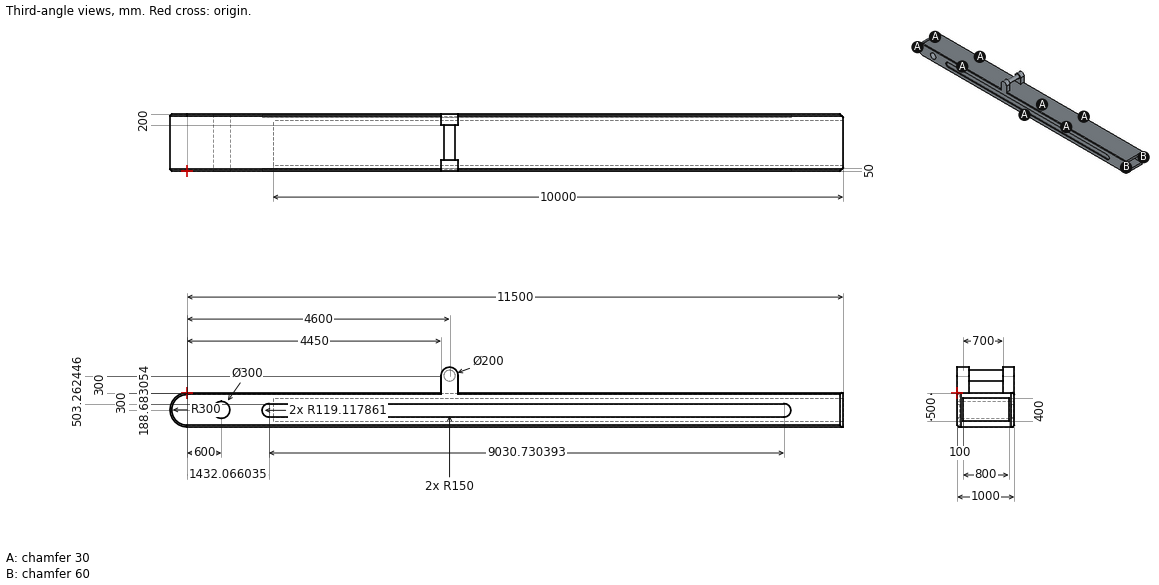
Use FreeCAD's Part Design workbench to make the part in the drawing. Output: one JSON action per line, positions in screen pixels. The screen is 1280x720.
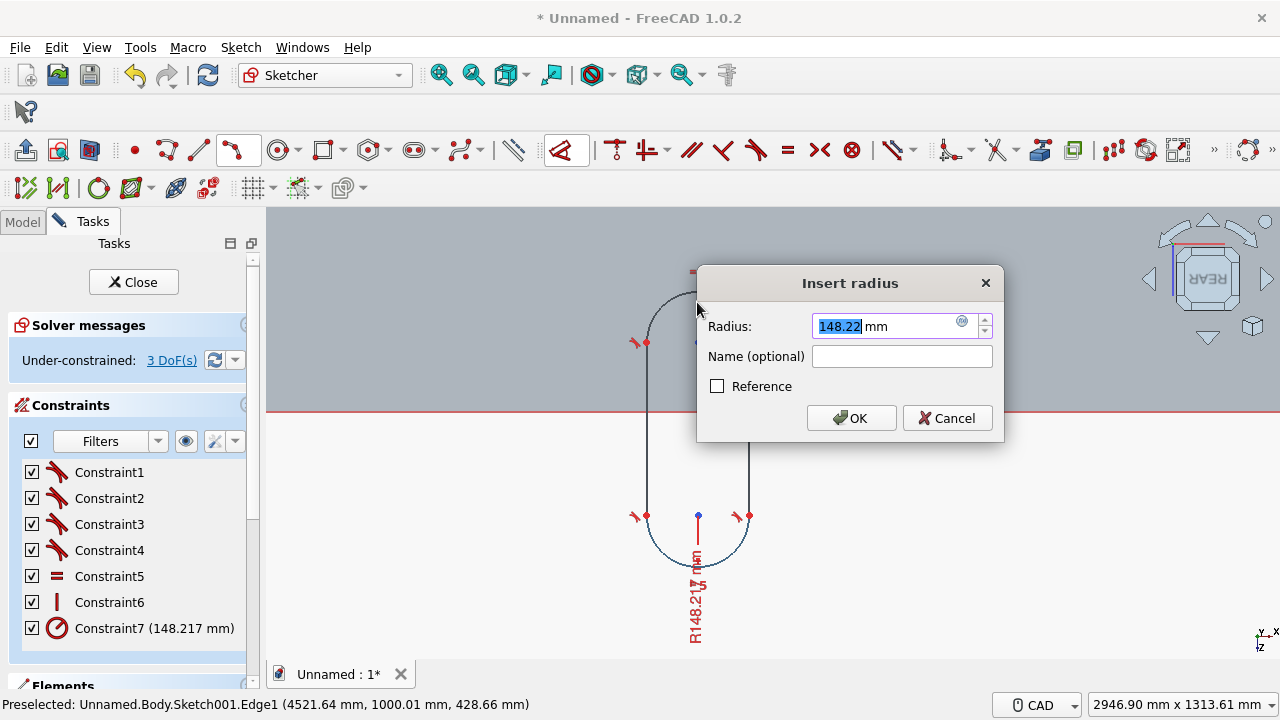
{"action": "type", "text": "150"}
{"action": "key", "text": "Return"}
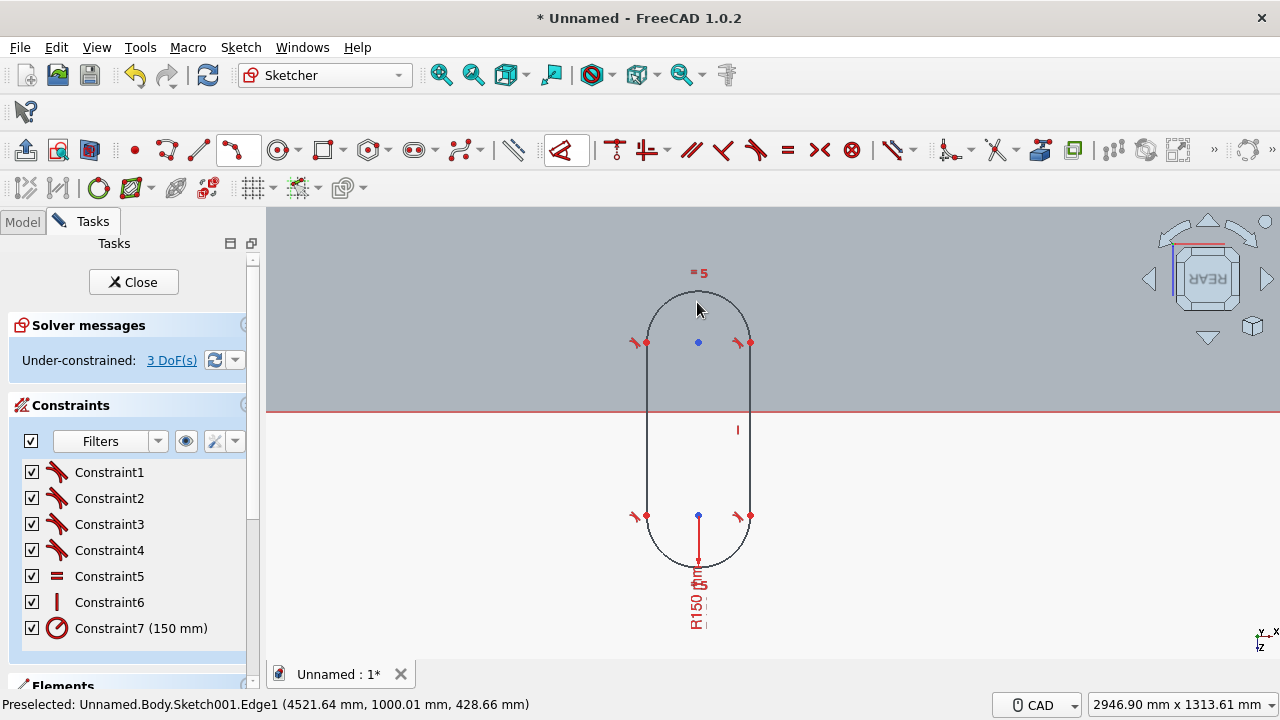
{"action": "left_click", "coordinate": [647, 516]}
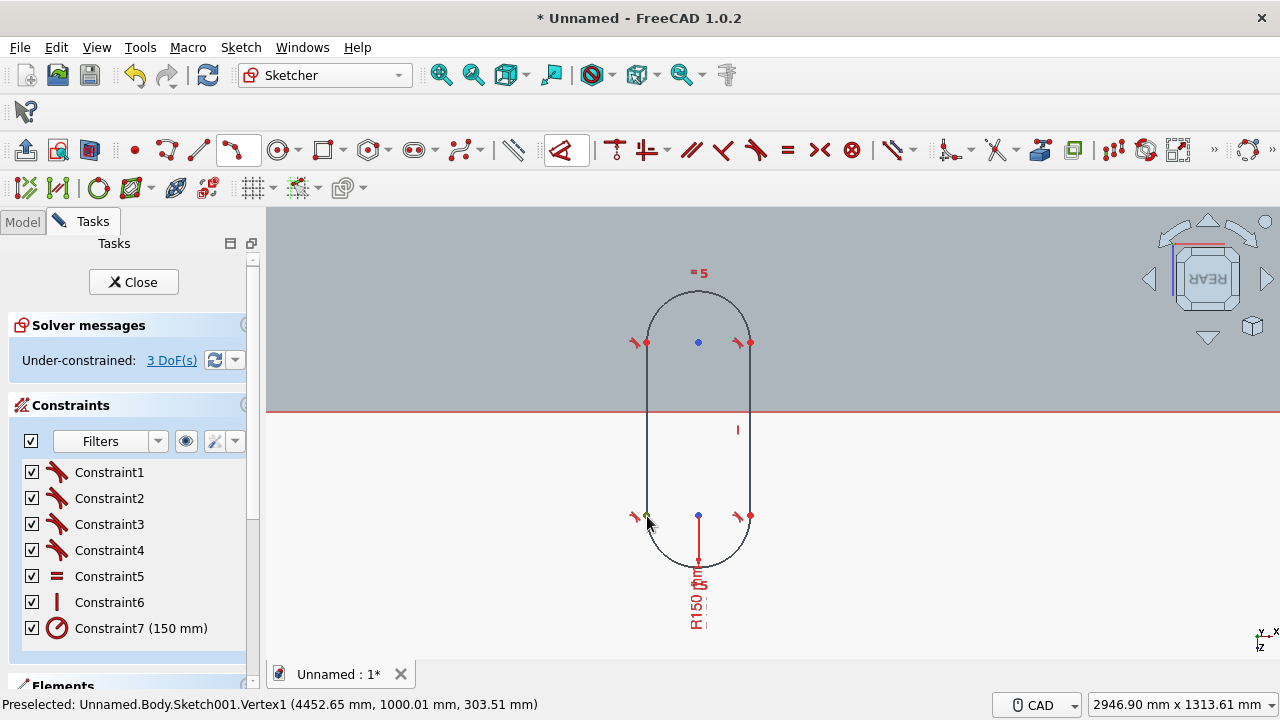
{"action": "left_click", "coordinate": [584, 150]}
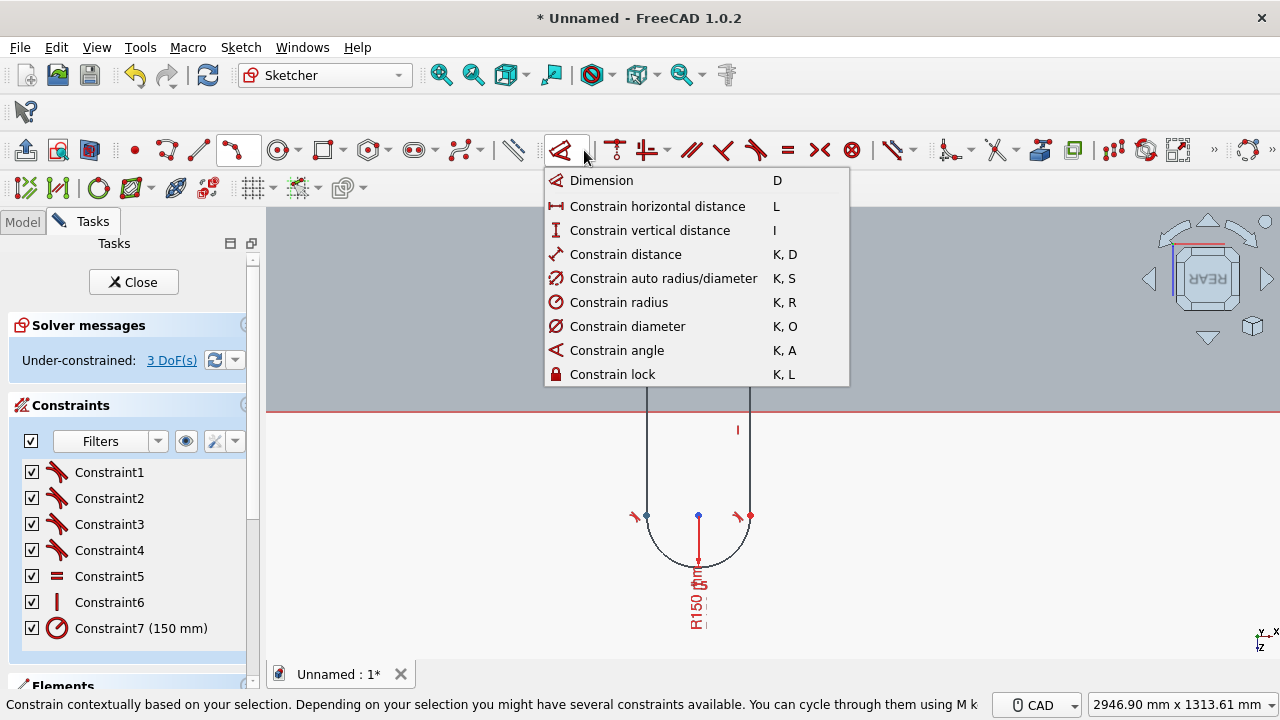
{"action": "left_click", "coordinate": [697, 230]}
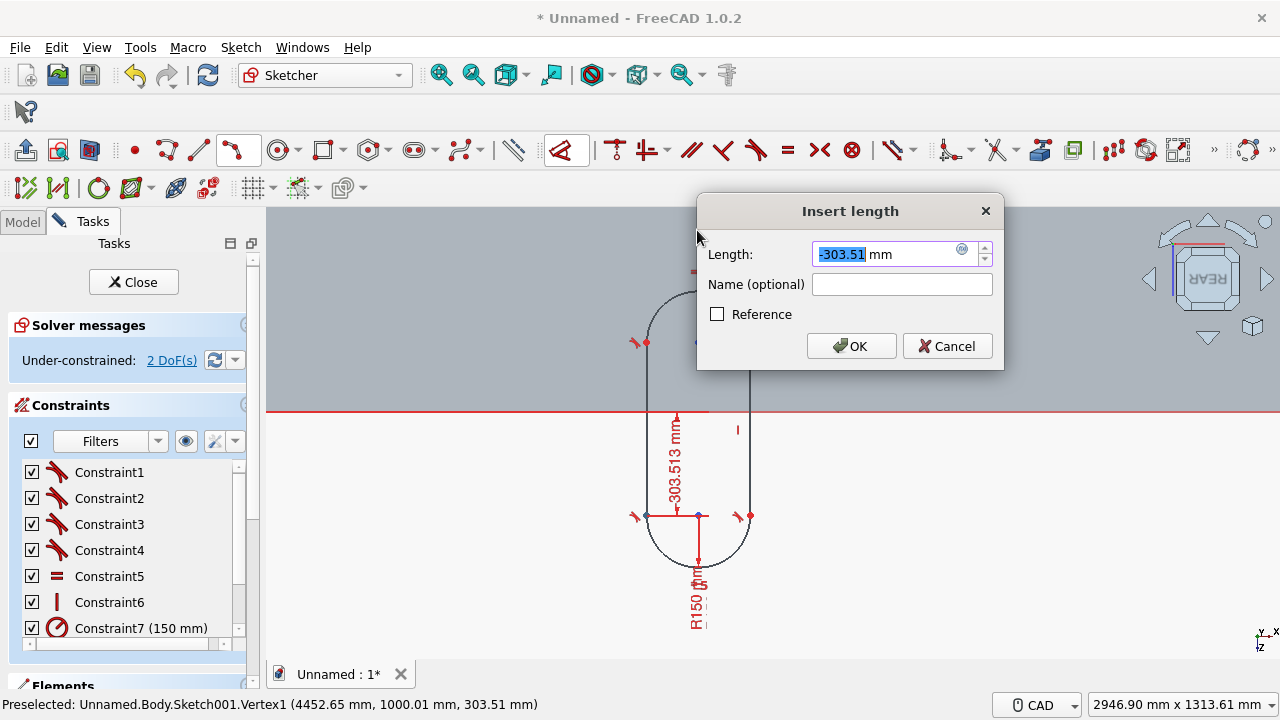
{"action": "type", "text": "-300"}
{"action": "key", "text": "Return"}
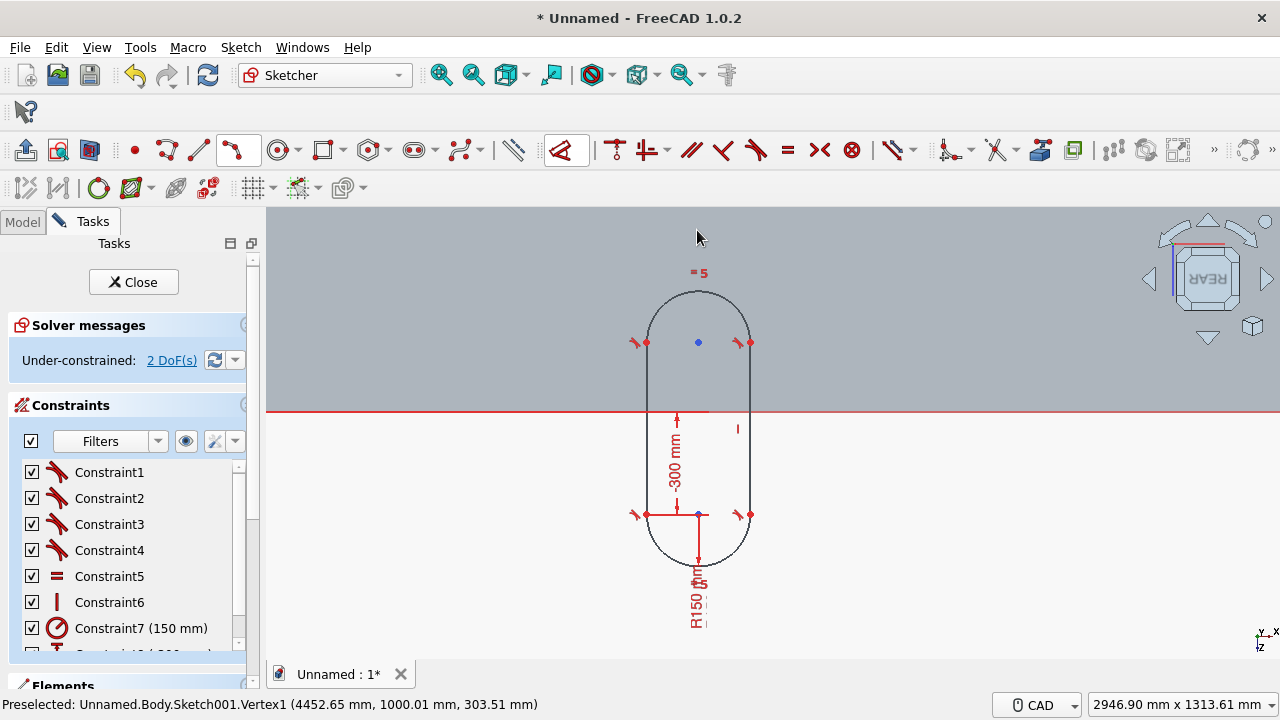
{"action": "left_click", "coordinate": [647, 515]}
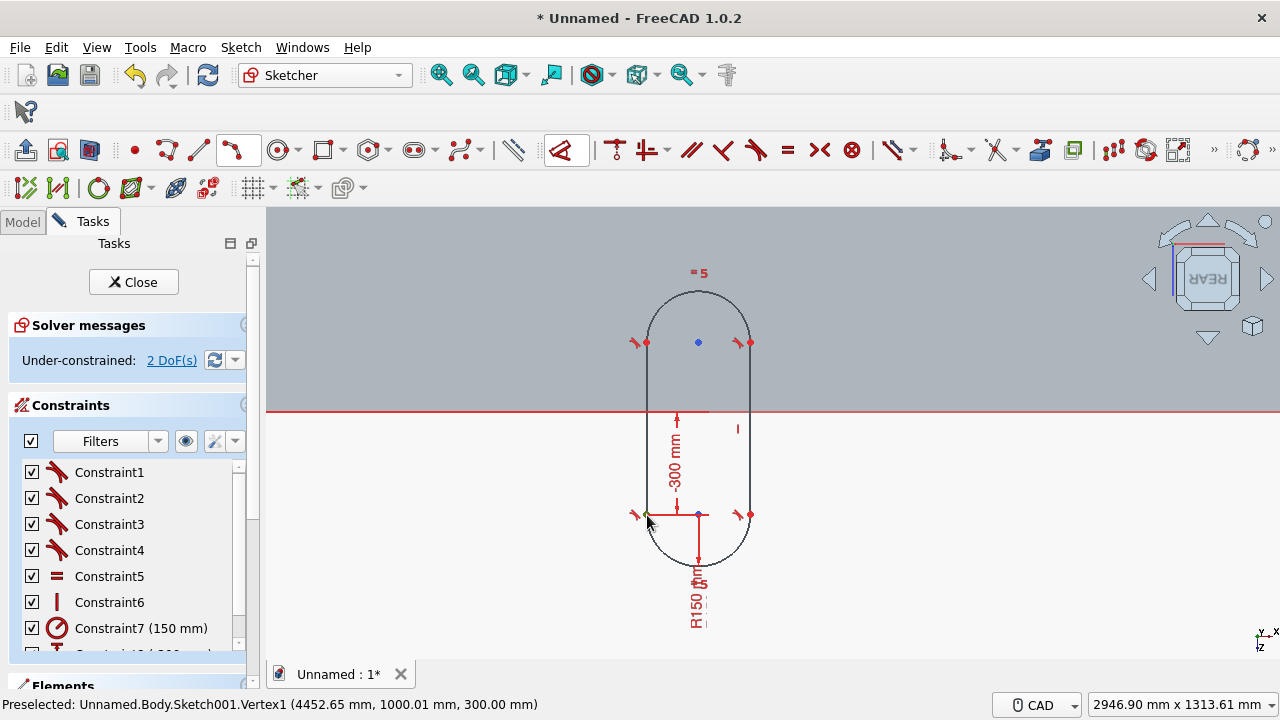
{"action": "key", "text": "l"}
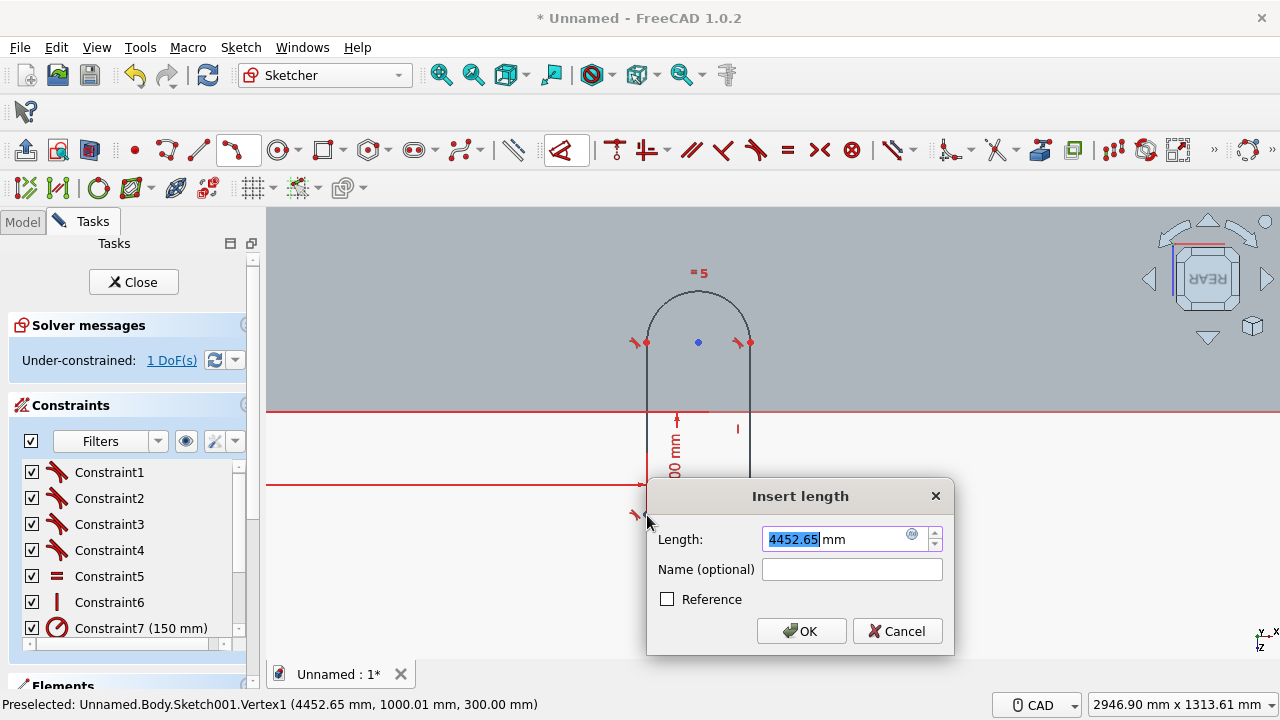
{"action": "type", "text": "4450"}
{"action": "key", "text": "Return"}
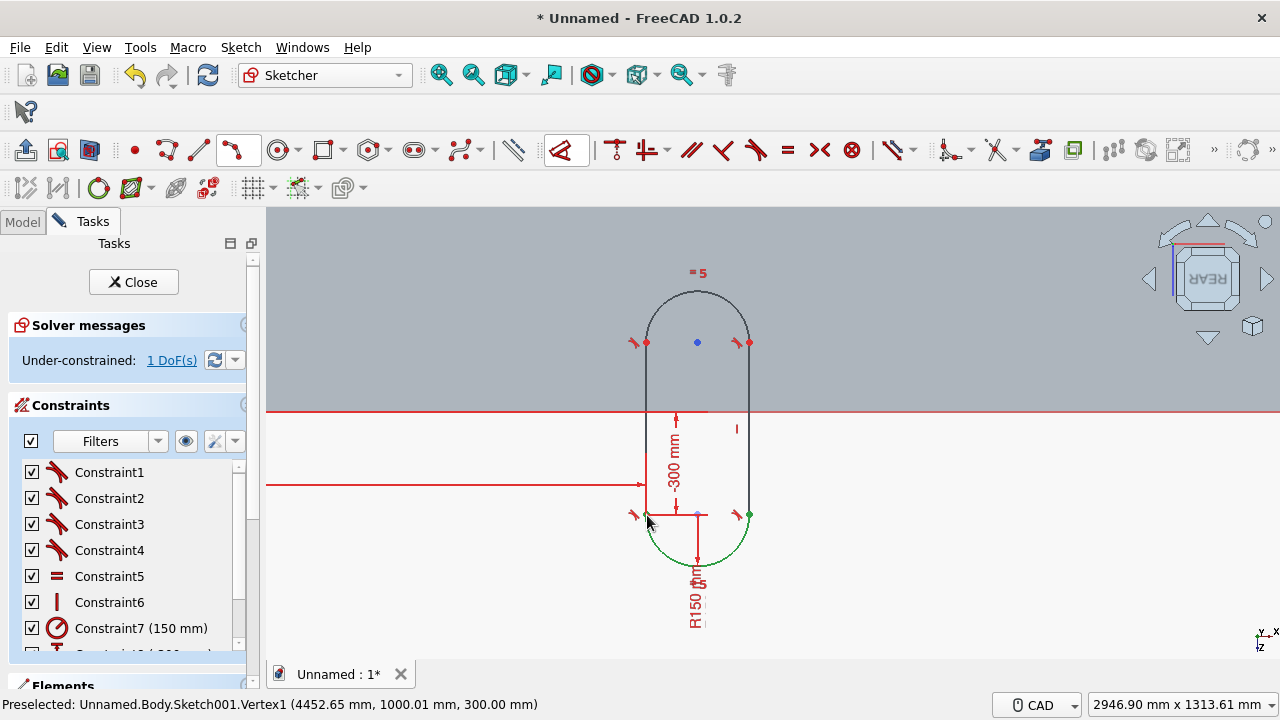
{"action": "left_click", "coordinate": [646, 463]}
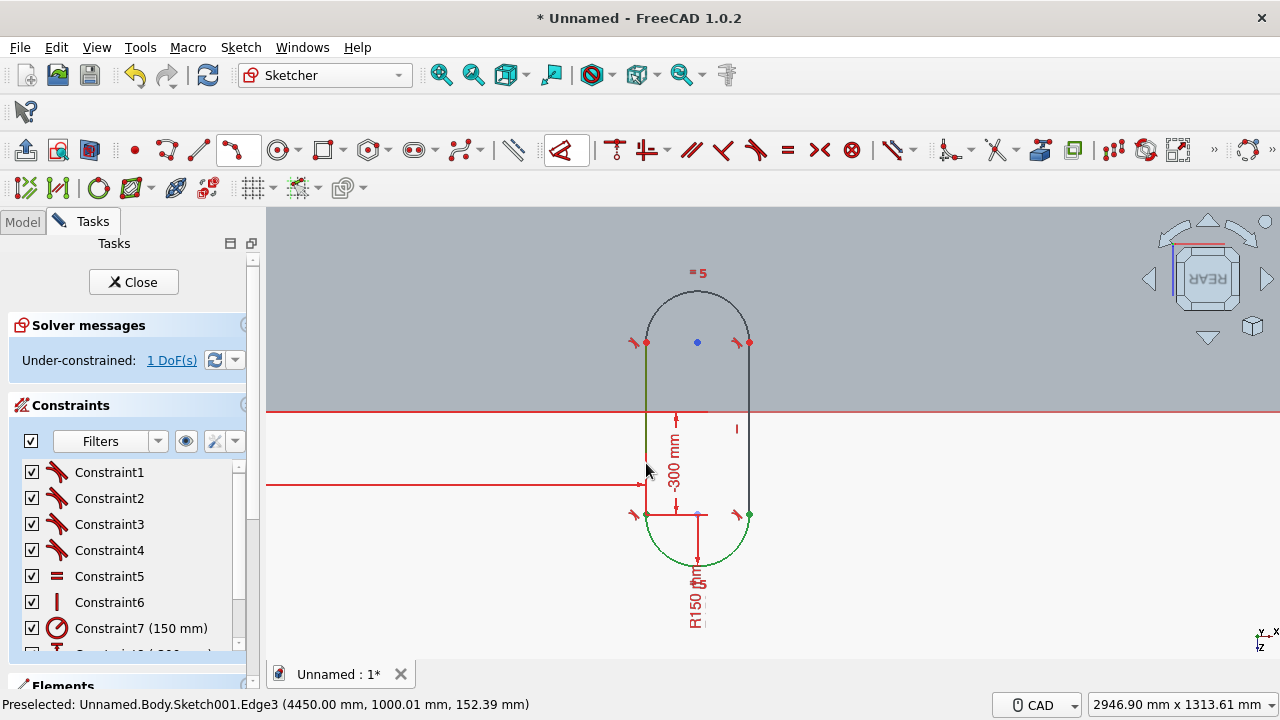
{"action": "left_click", "coordinate": [584, 150]}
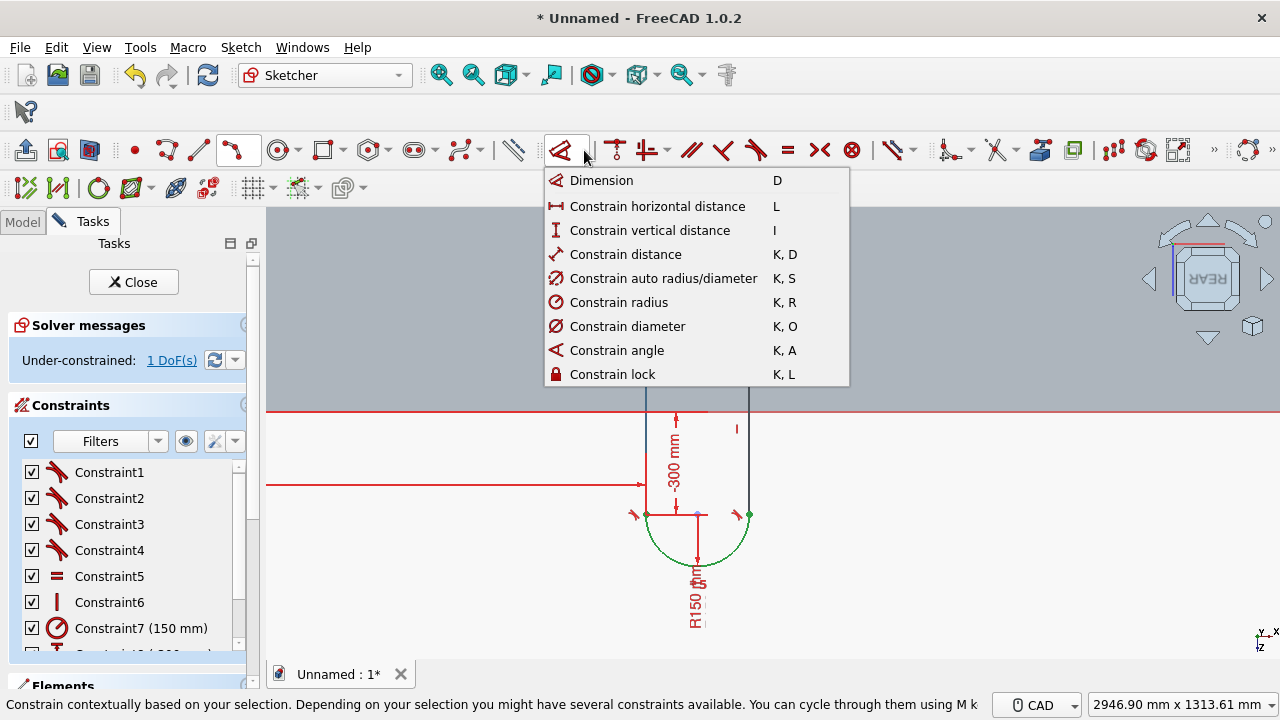
{"action": "left_click", "coordinate": [697, 230]}